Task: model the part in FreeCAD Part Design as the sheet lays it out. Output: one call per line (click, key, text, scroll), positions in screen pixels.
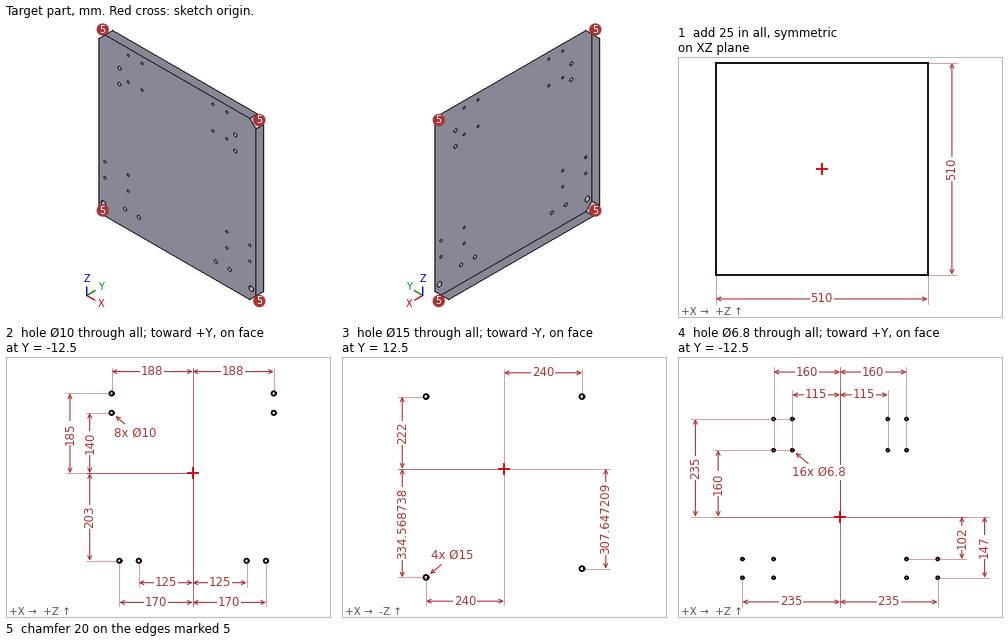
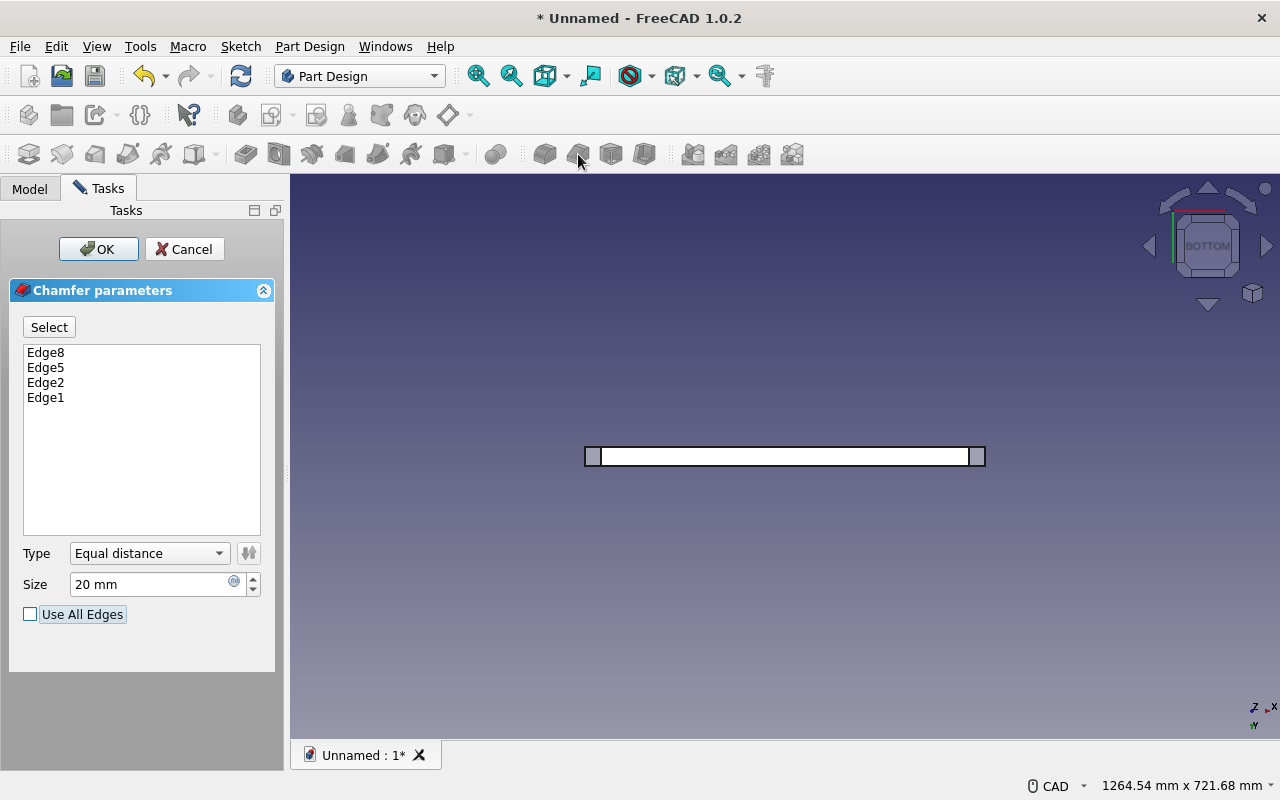
click(99, 249)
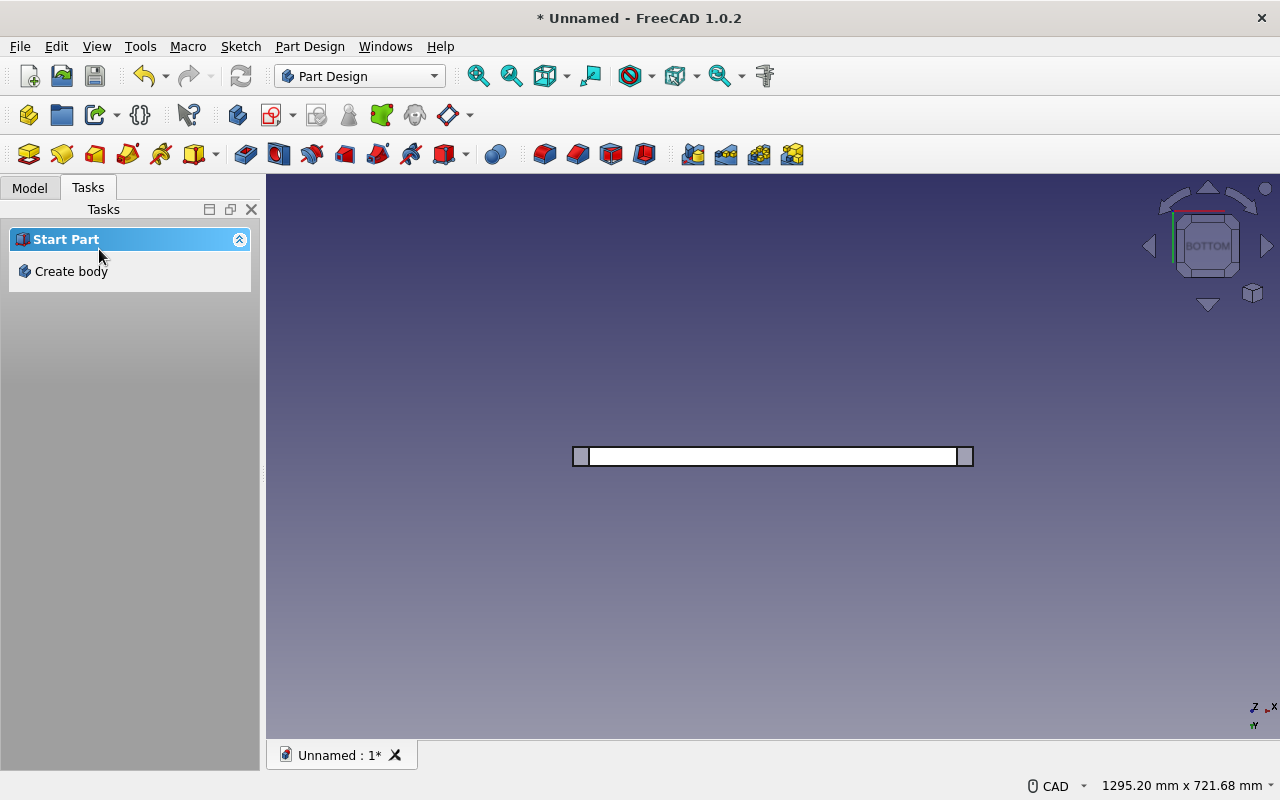
key(0)